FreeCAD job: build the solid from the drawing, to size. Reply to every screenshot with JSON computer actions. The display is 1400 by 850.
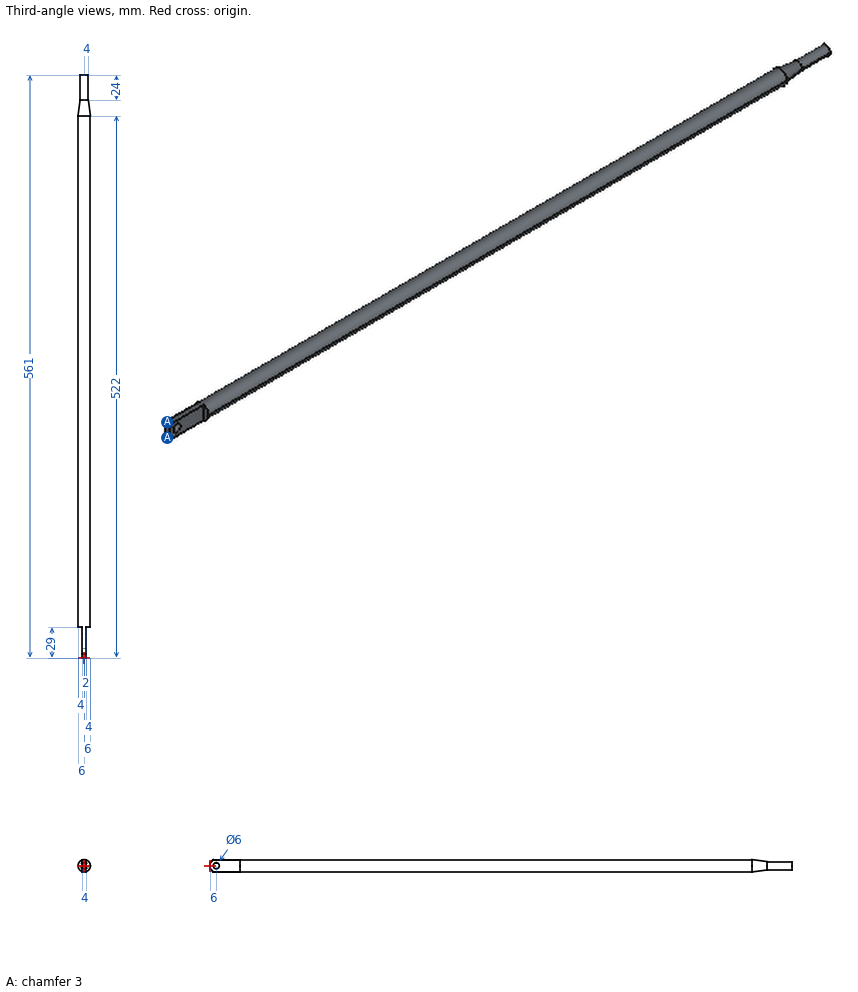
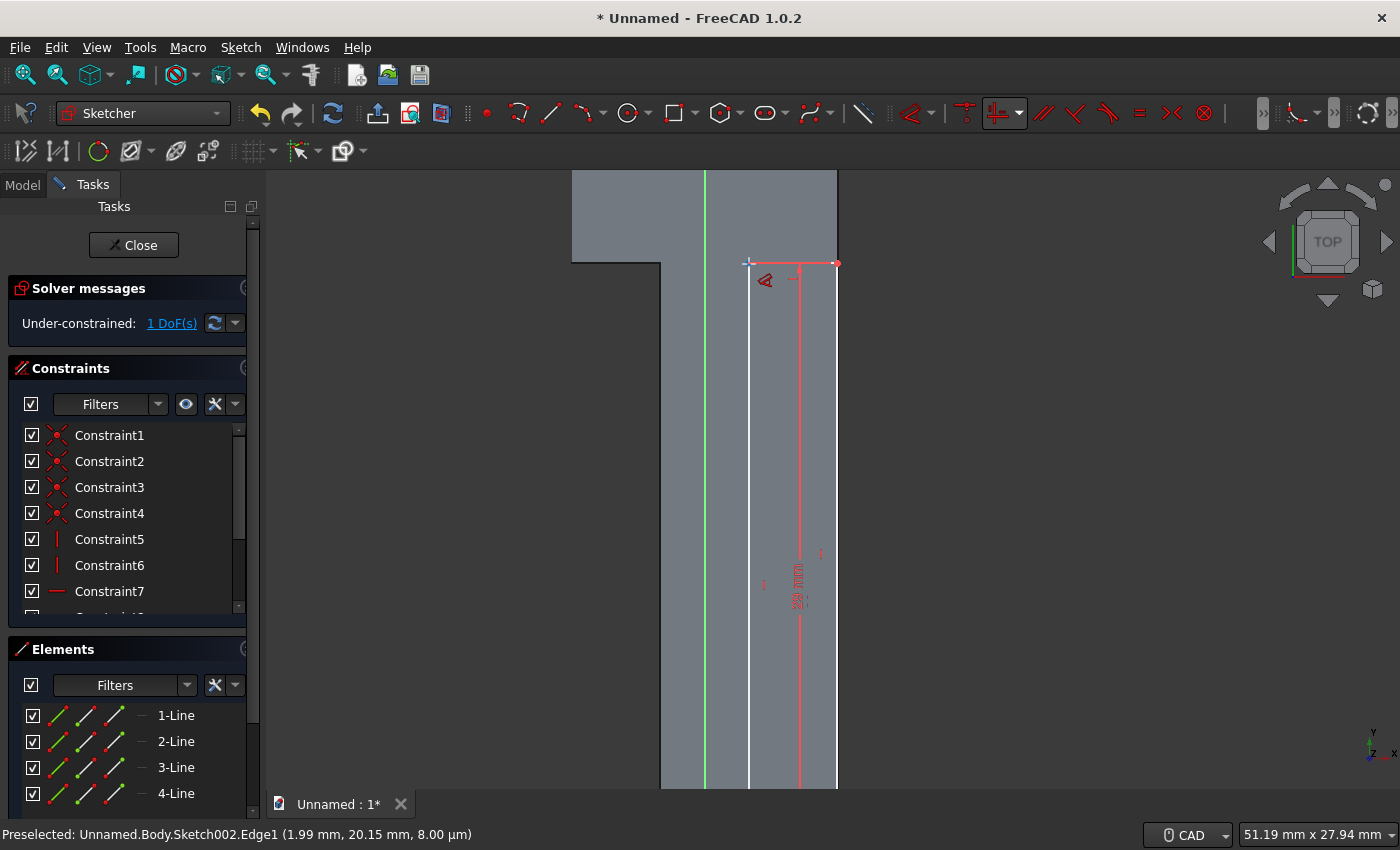
{"action": "left_click", "coordinate": [749, 263]}
{"action": "left_click", "coordinate": [727, 229]}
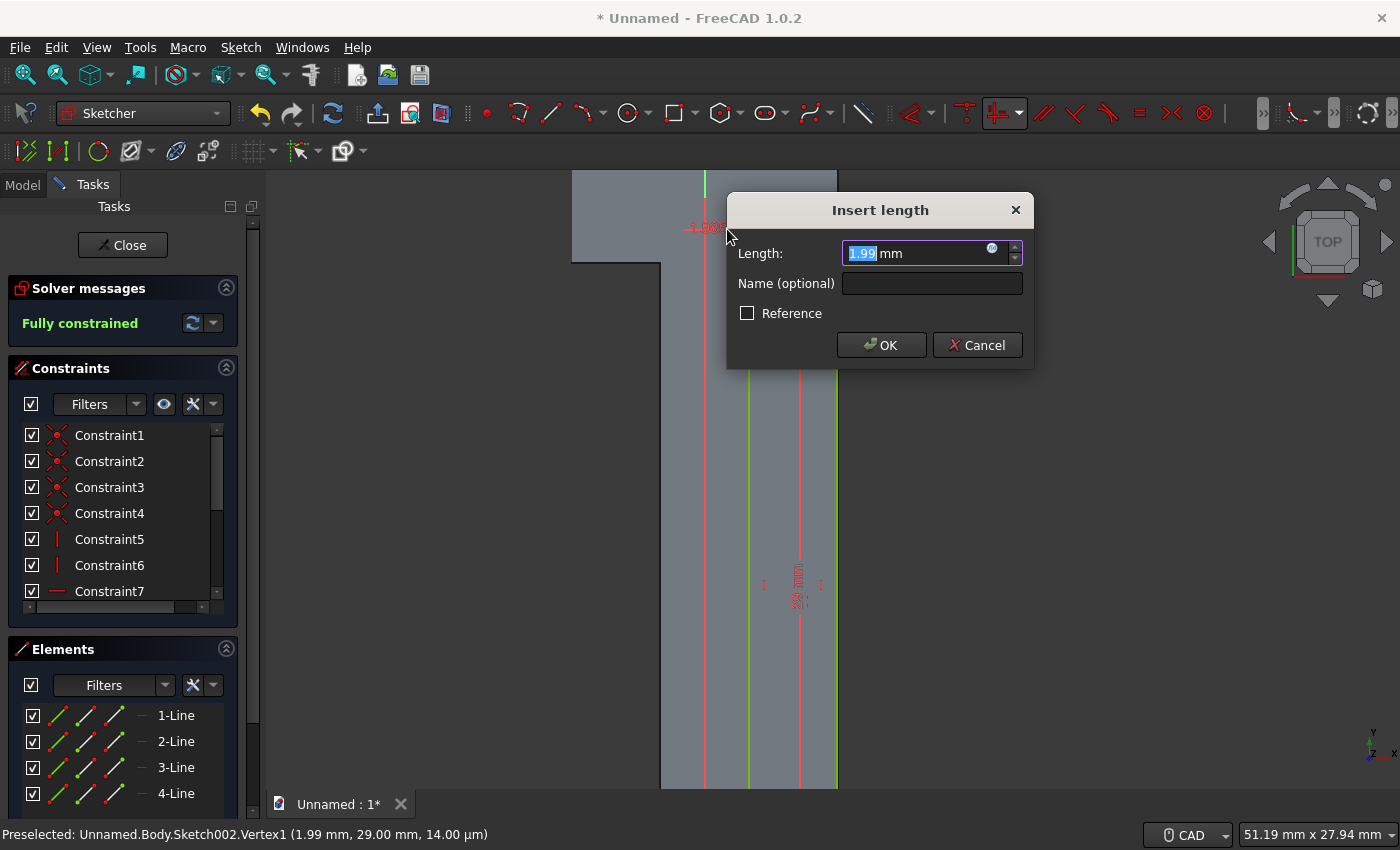
{"action": "type", "text": "2"}
{"action": "key", "text": "Return"}
{"action": "key", "text": "Escape"}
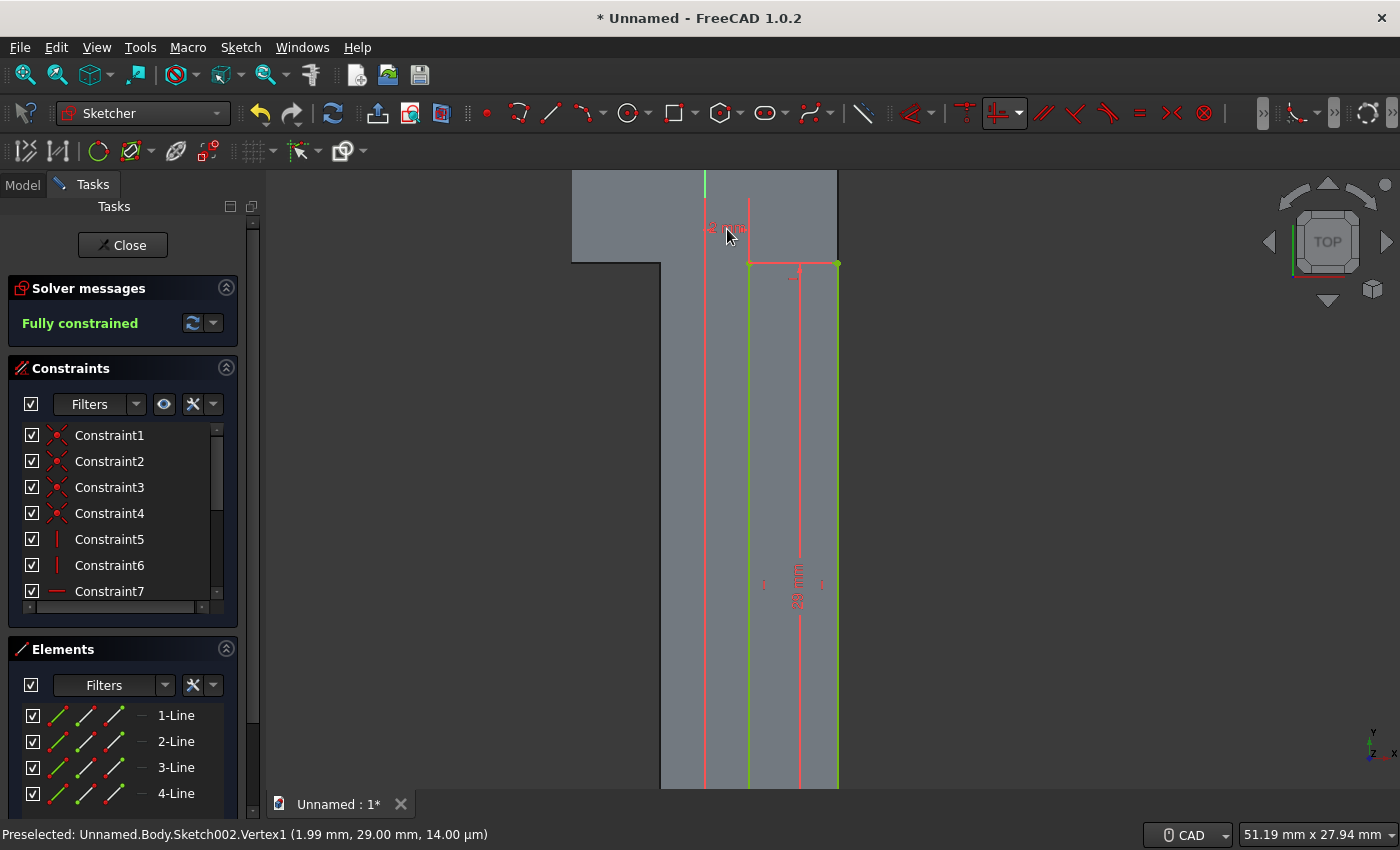
{"action": "left_click", "coordinate": [123, 245]}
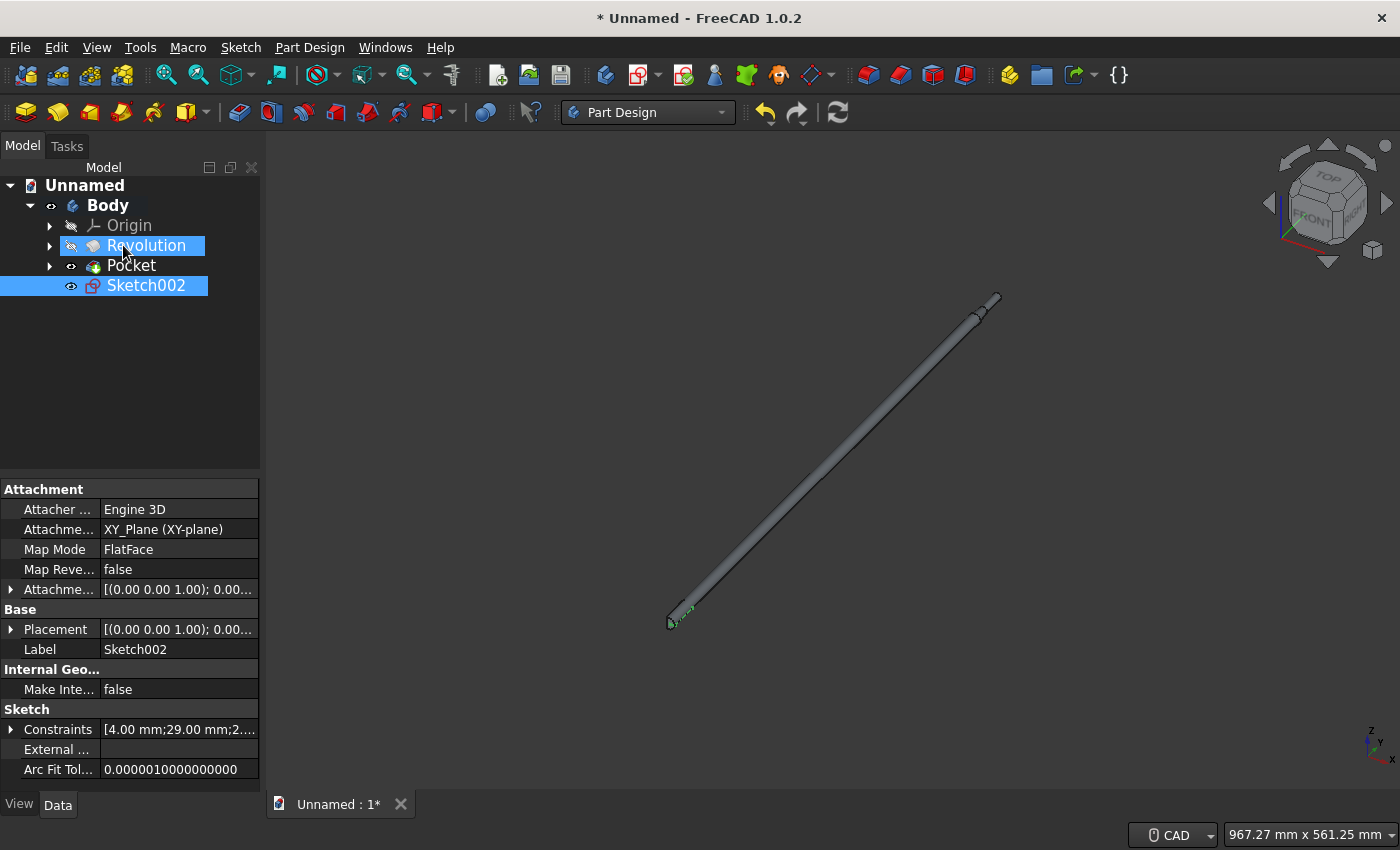
{"action": "left_click", "coordinate": [240, 112]}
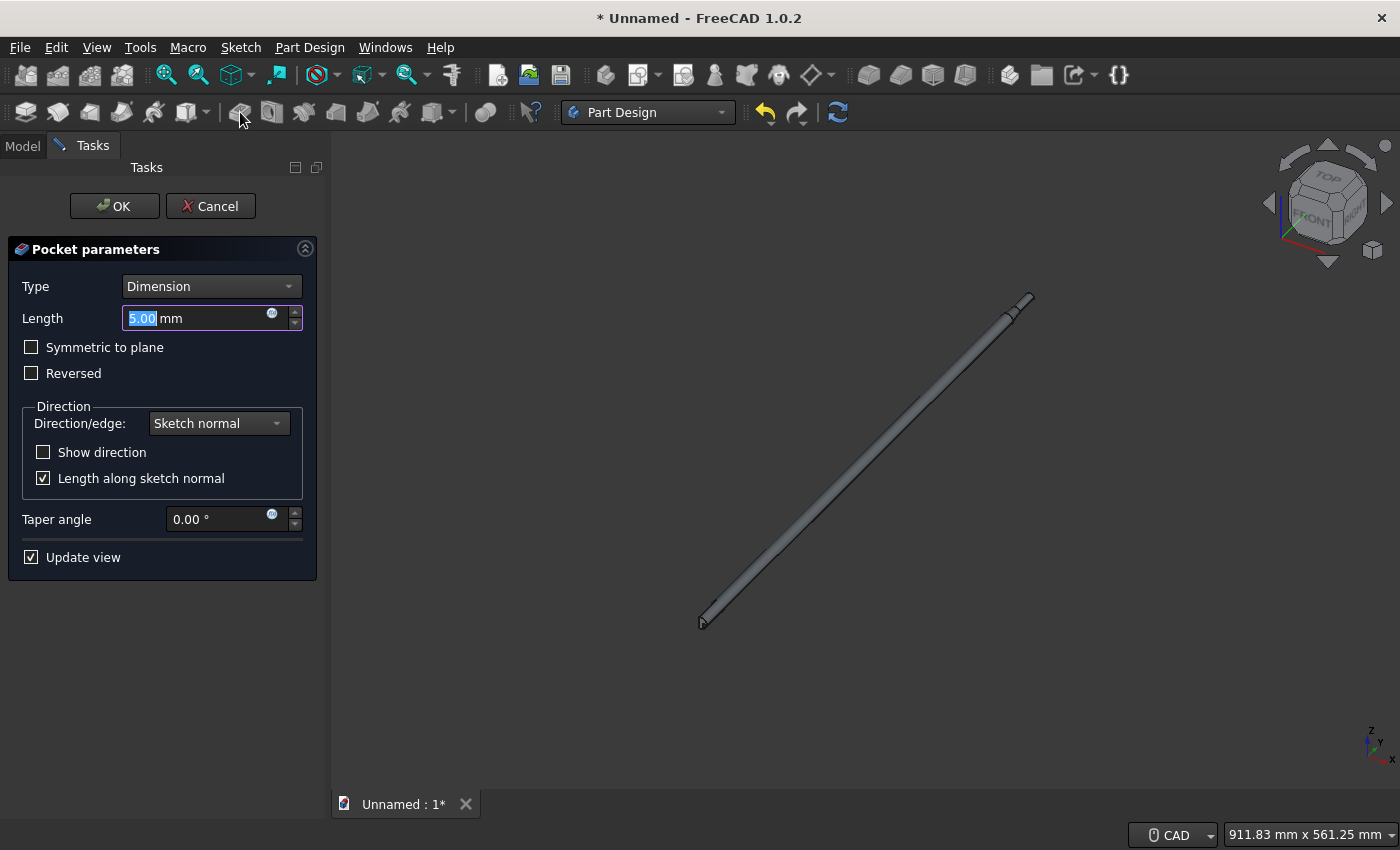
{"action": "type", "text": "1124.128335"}
{"action": "key", "text": "Tab"}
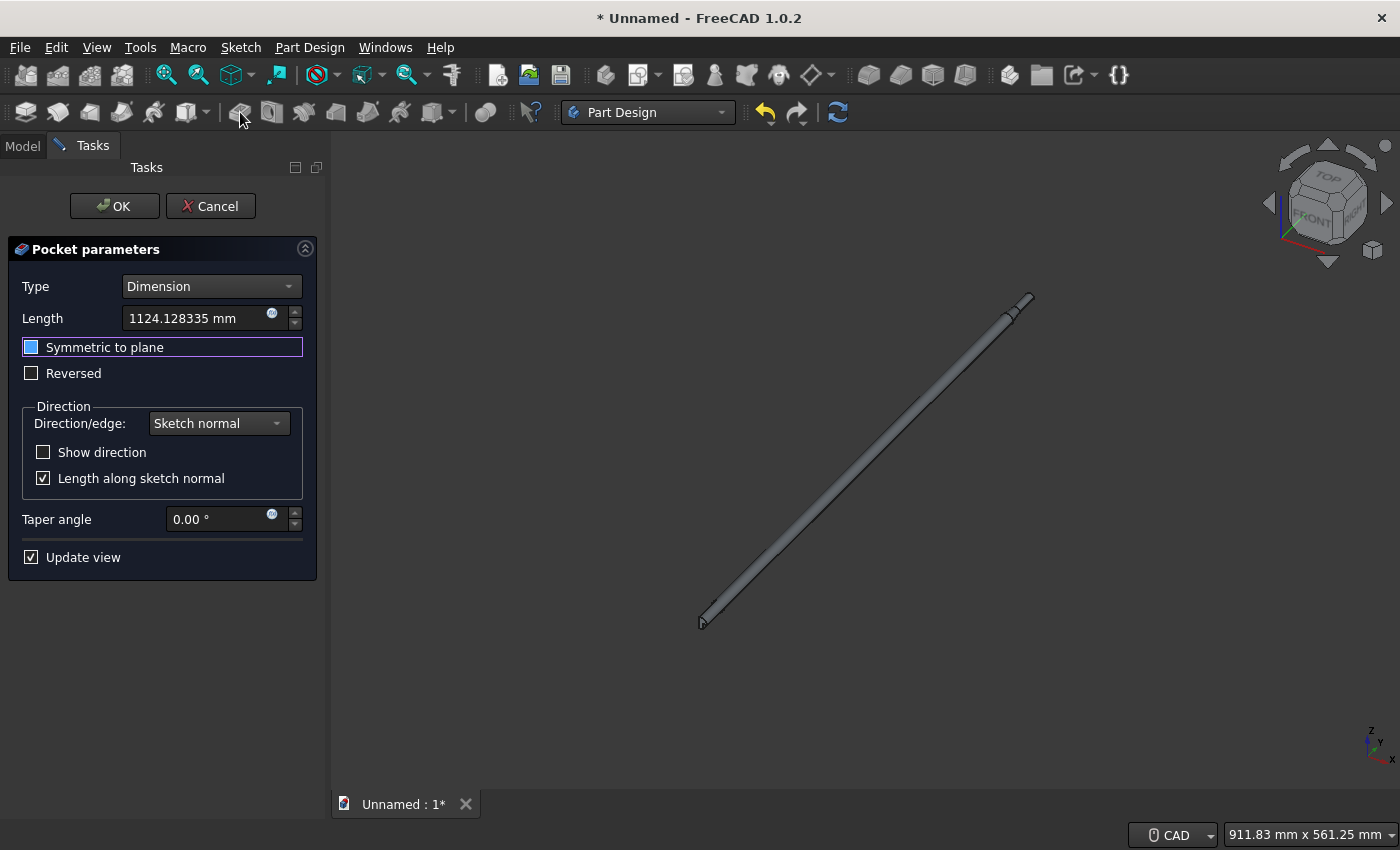
{"action": "left_click", "coordinate": [30, 347]}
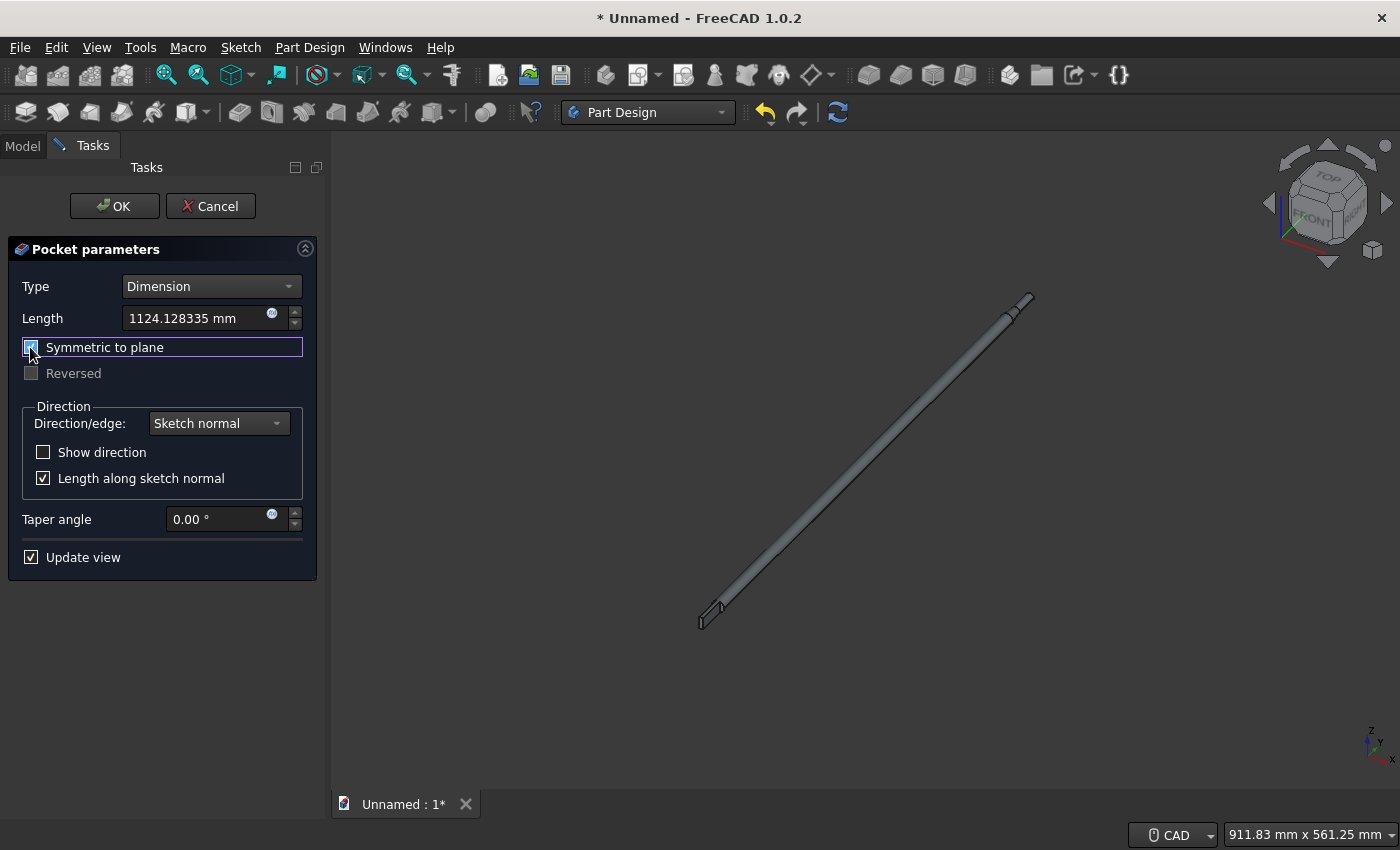
{"action": "left_click", "coordinate": [115, 206]}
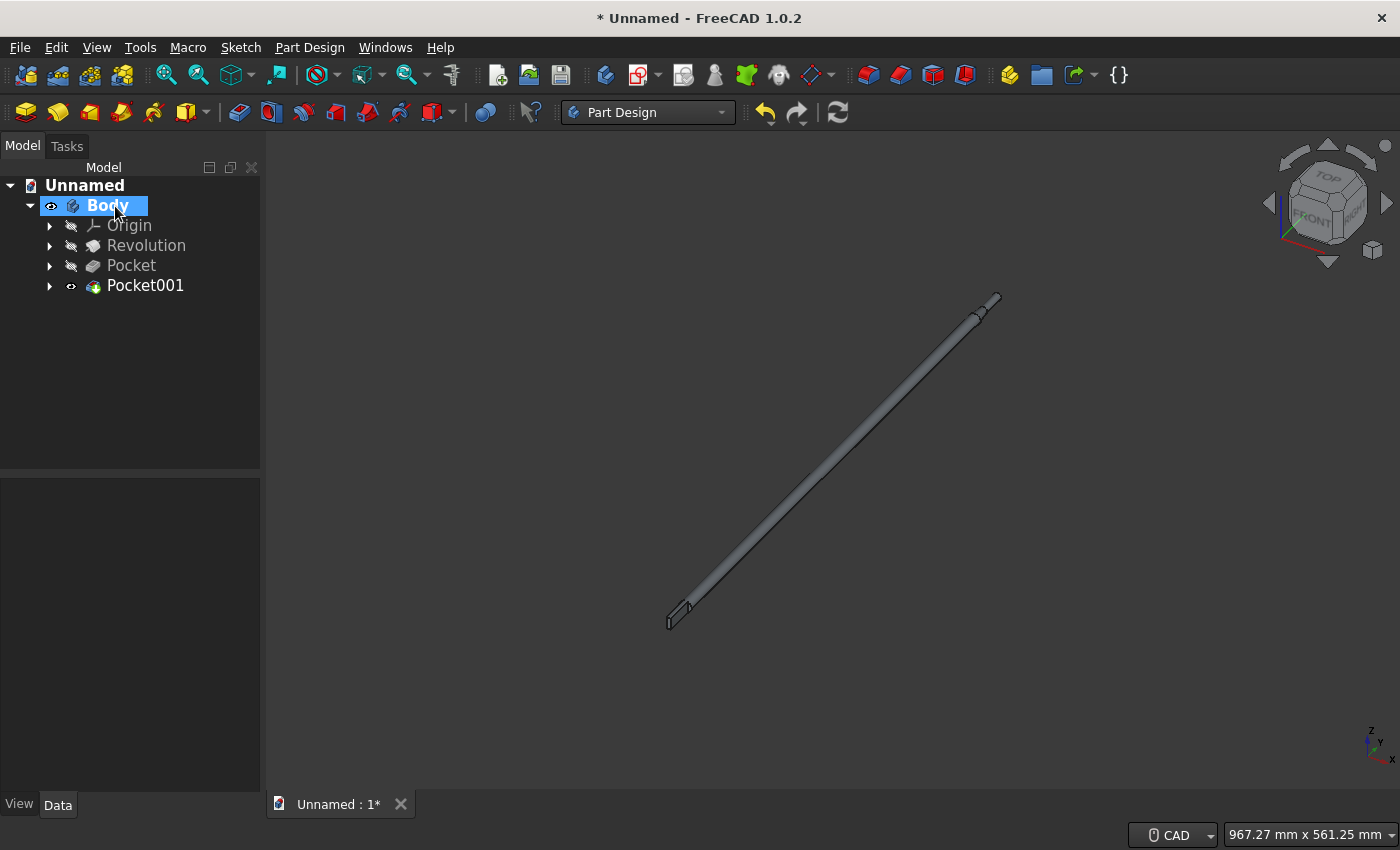
{"action": "scroll", "coordinate": [669, 628], "scroll_direction": "up", "scroll_amount": 11}